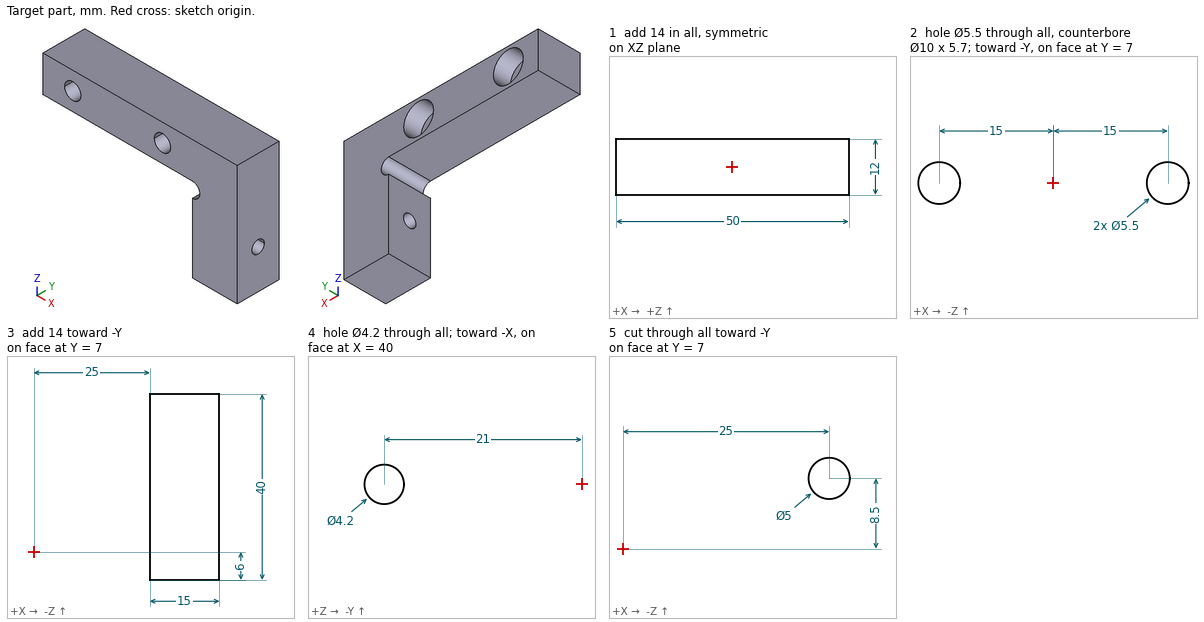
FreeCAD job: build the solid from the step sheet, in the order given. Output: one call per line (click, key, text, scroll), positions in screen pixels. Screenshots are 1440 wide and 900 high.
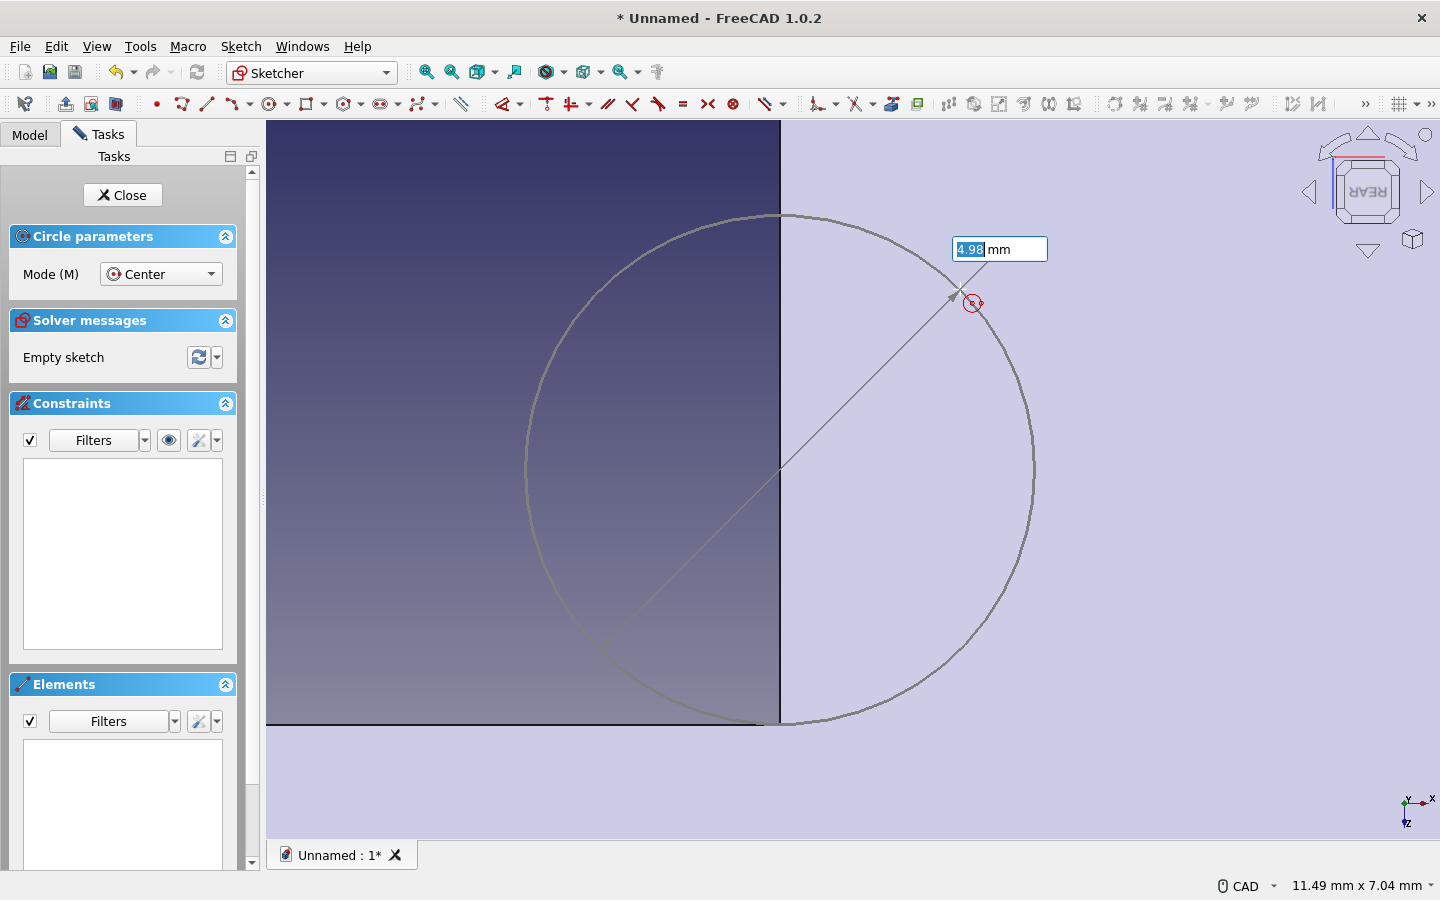
text(5)
key(Return)
key(Escape)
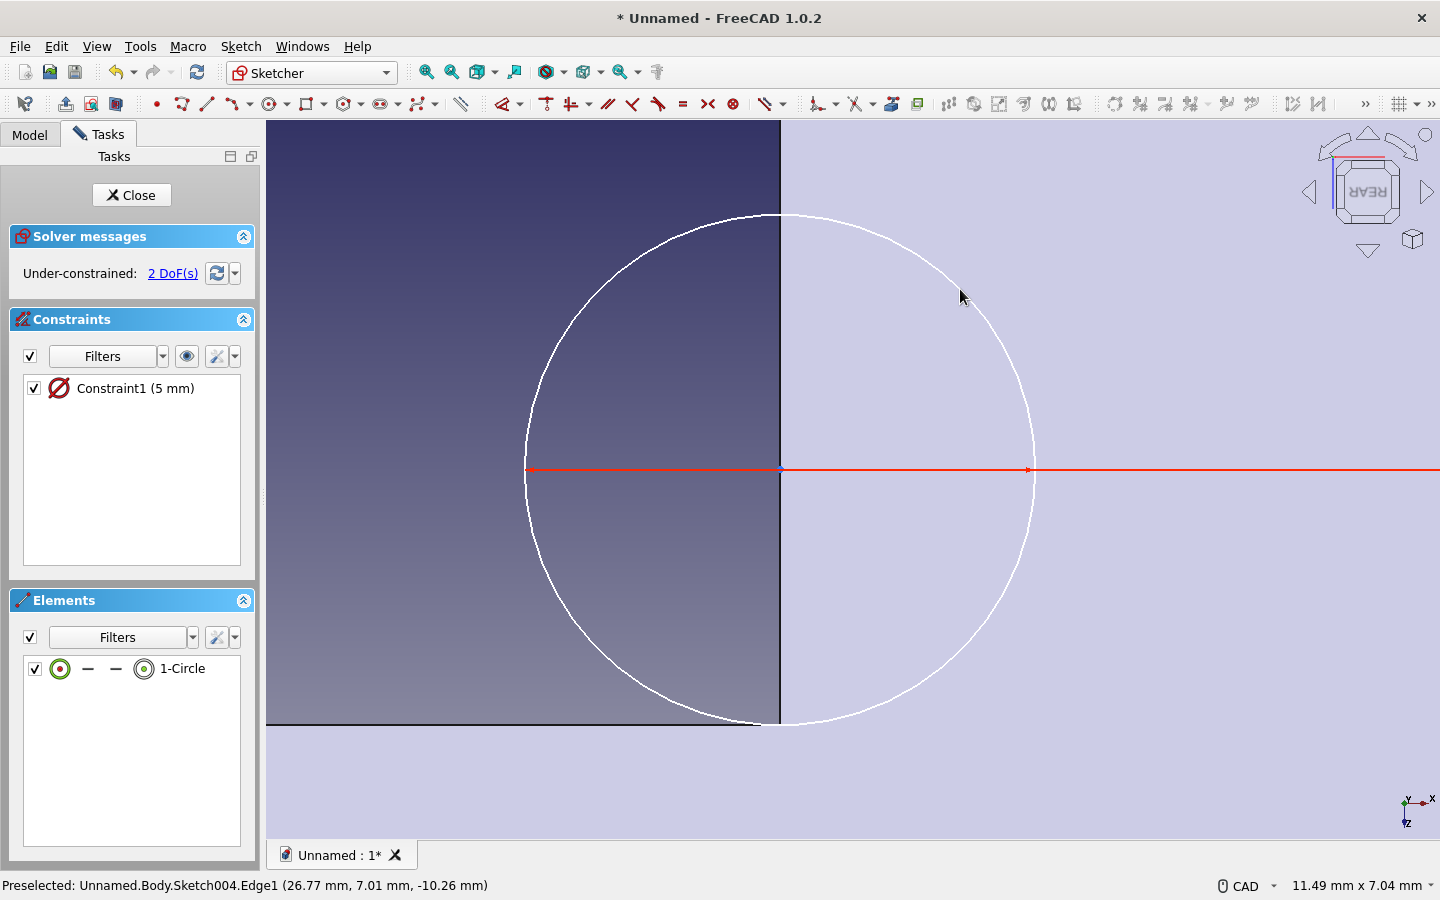
click(502, 104)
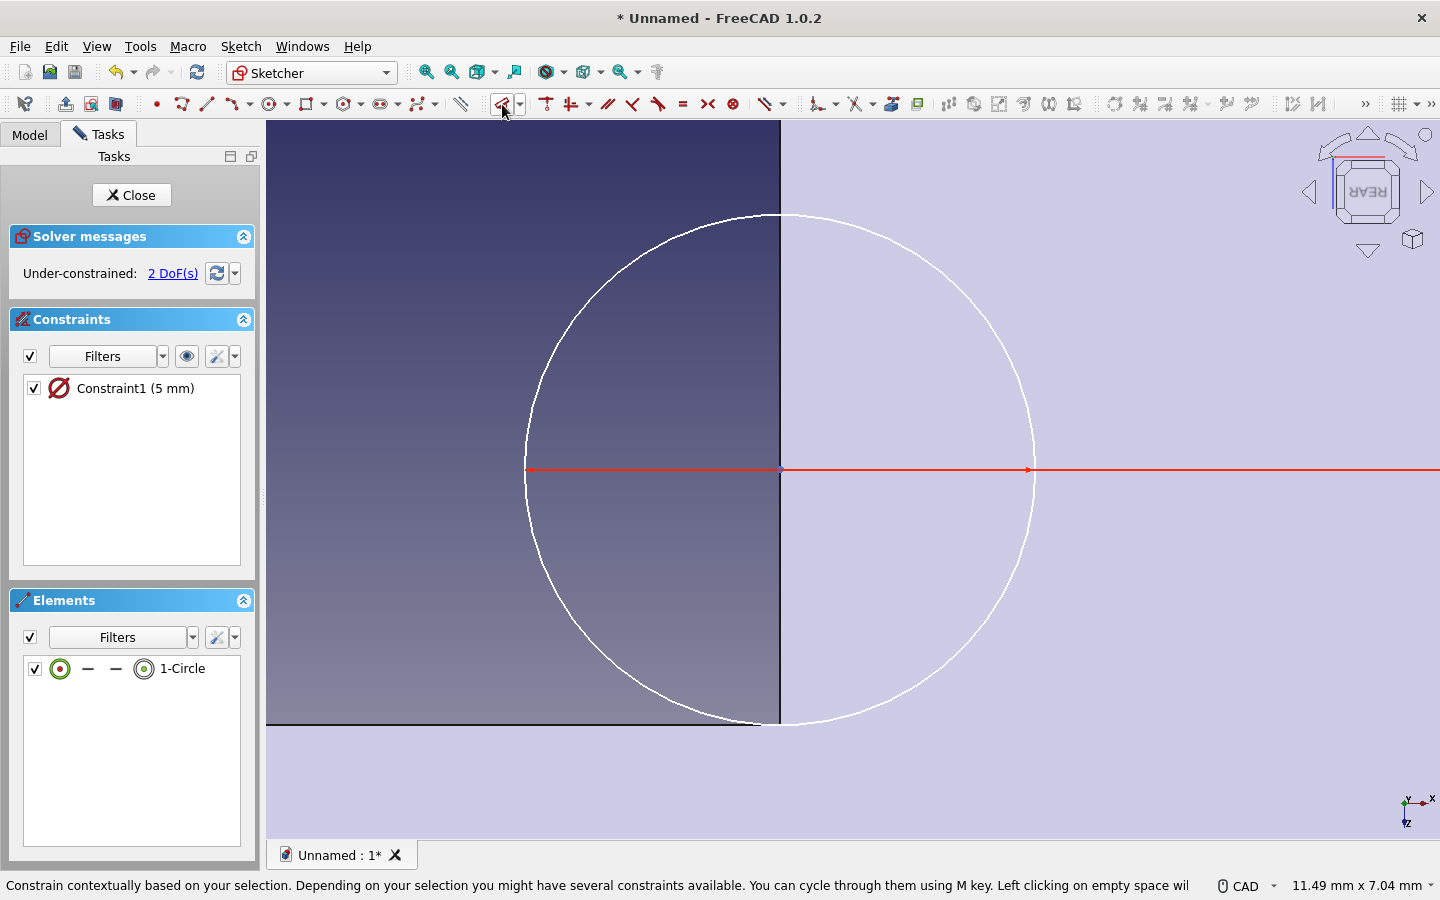
click(780, 470)
click(425, 436)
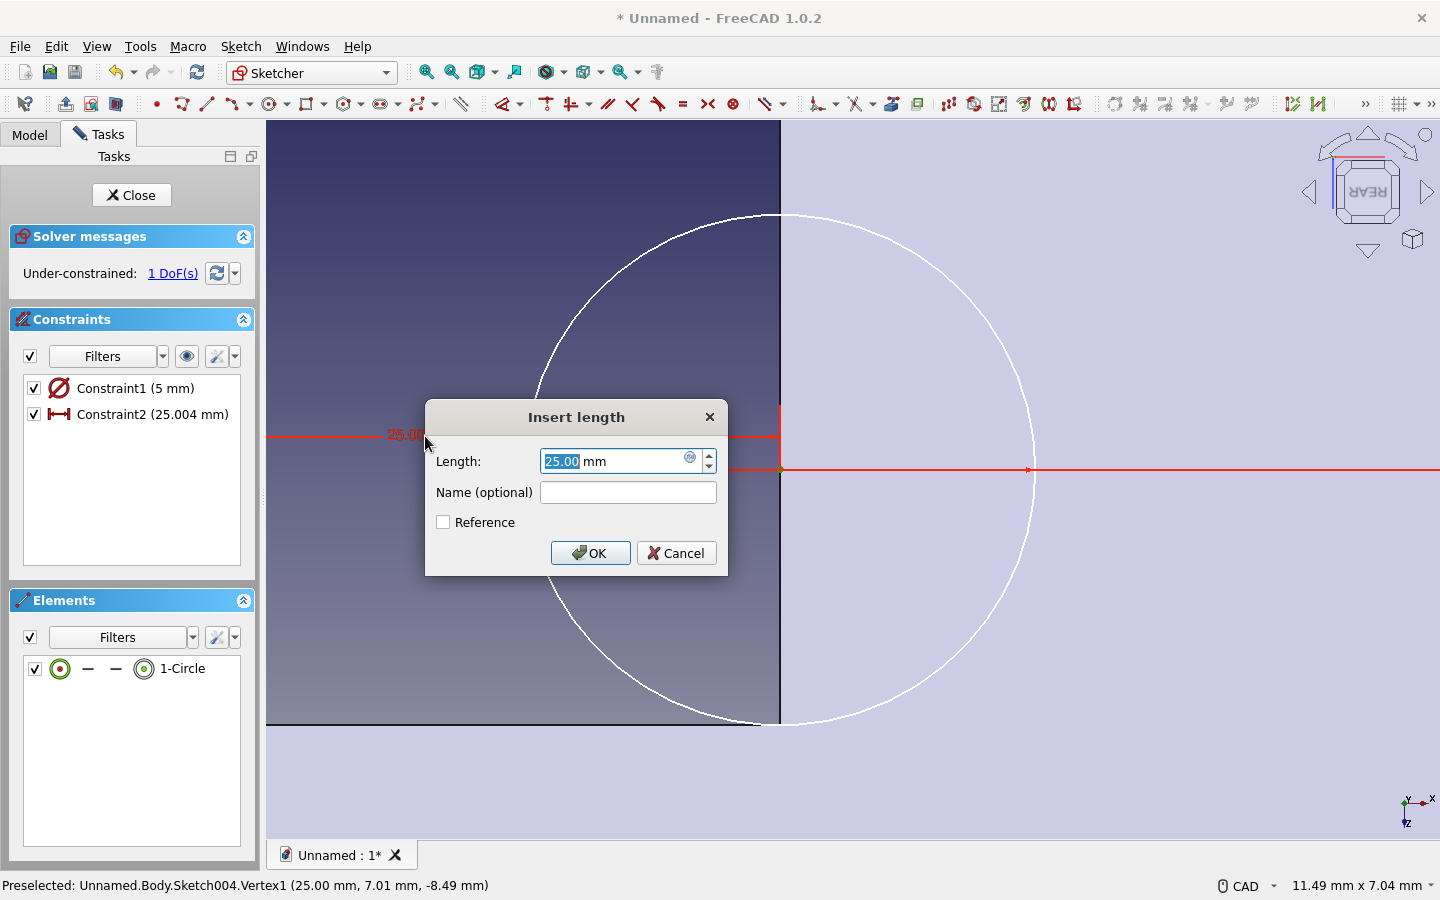
text(25)
key(Return)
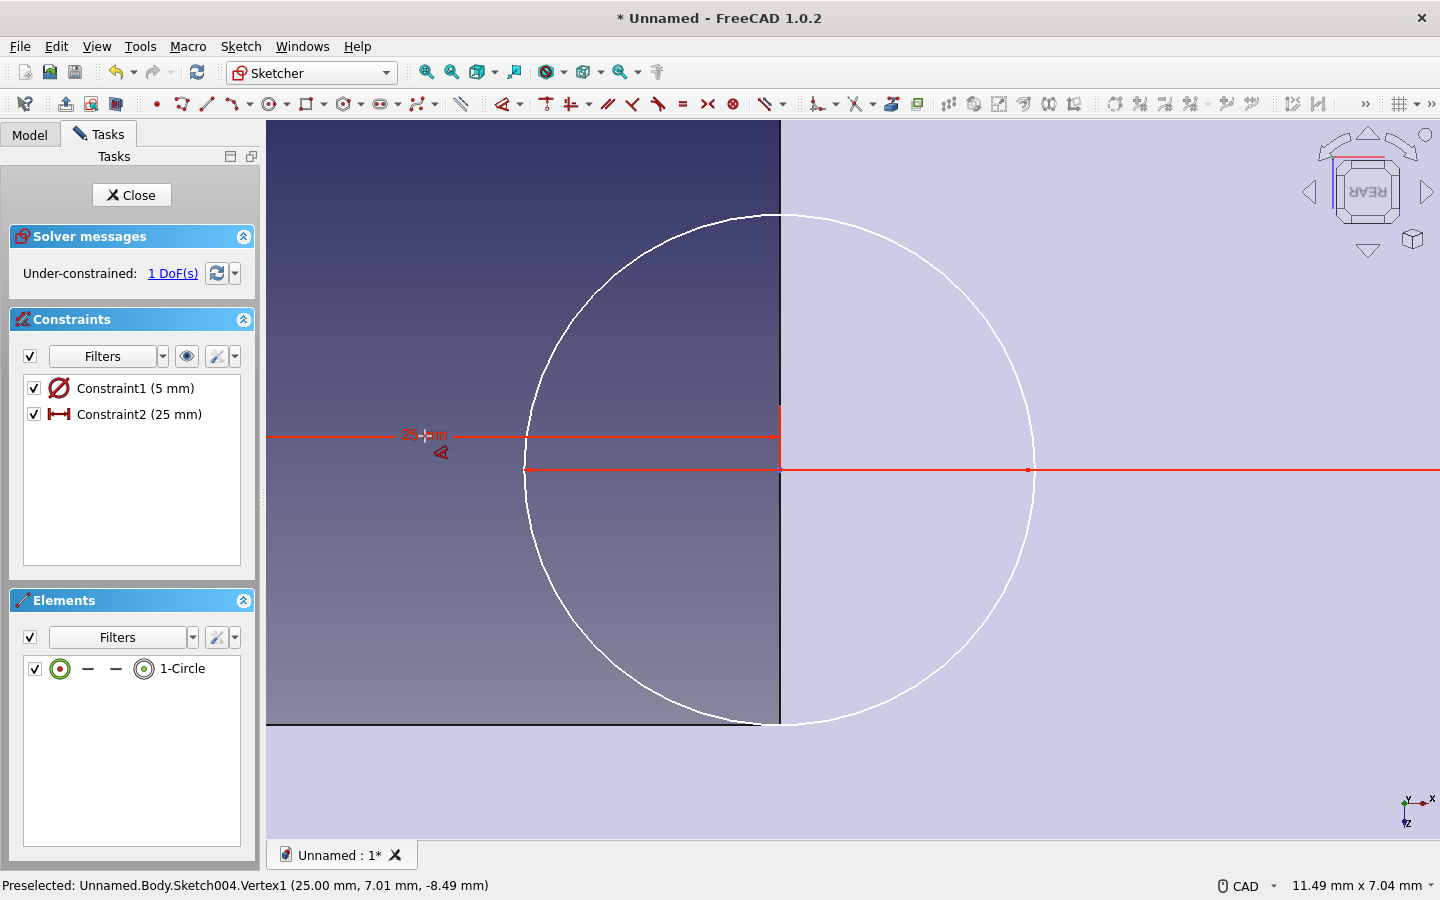
click(780, 470)
click(814, 641)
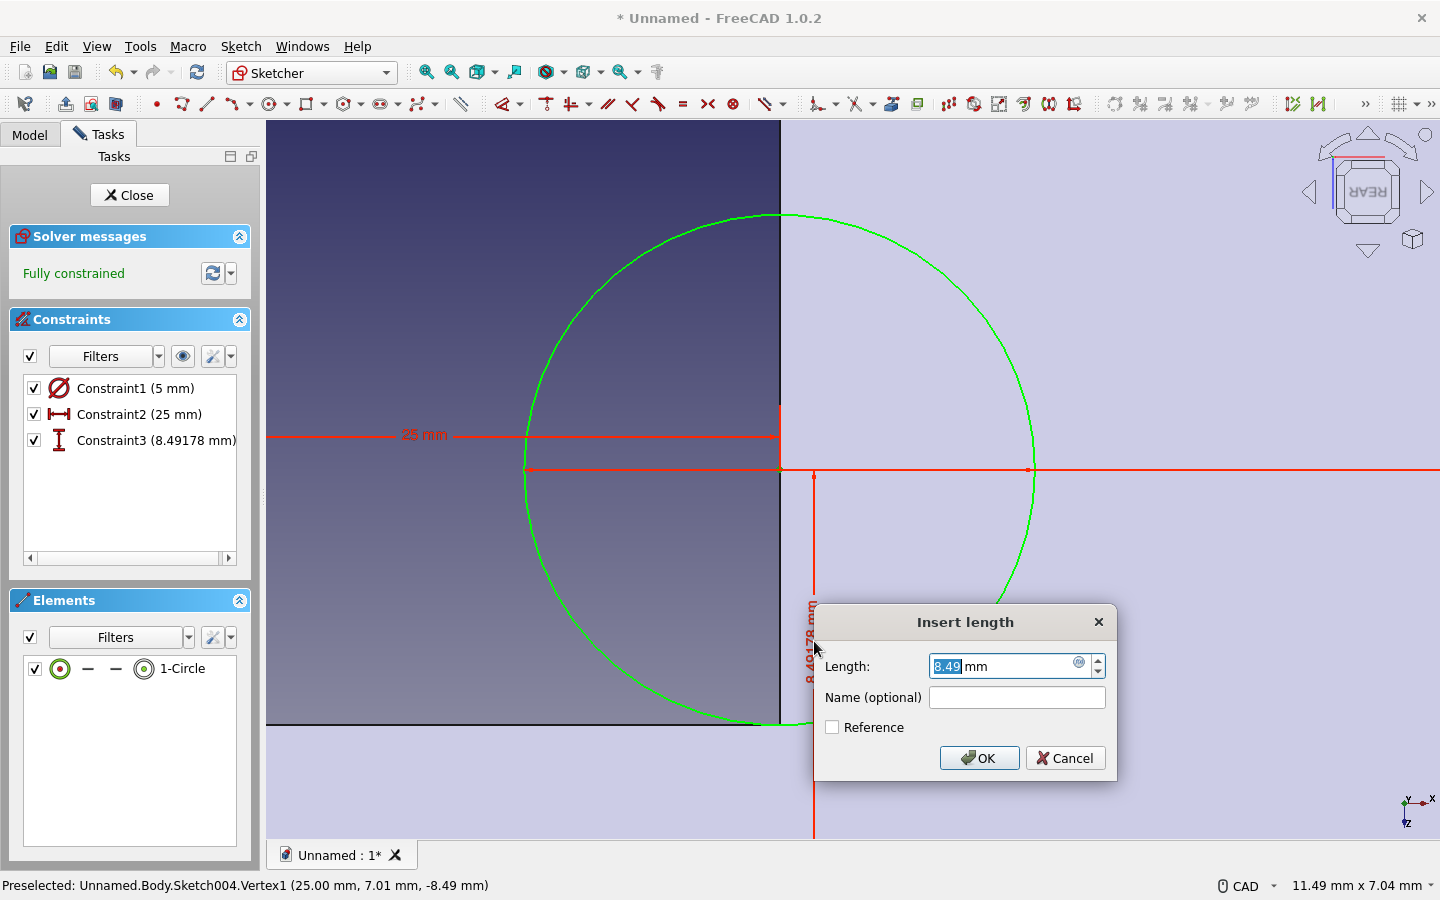
text(8.5)
key(Return)
key(Escape)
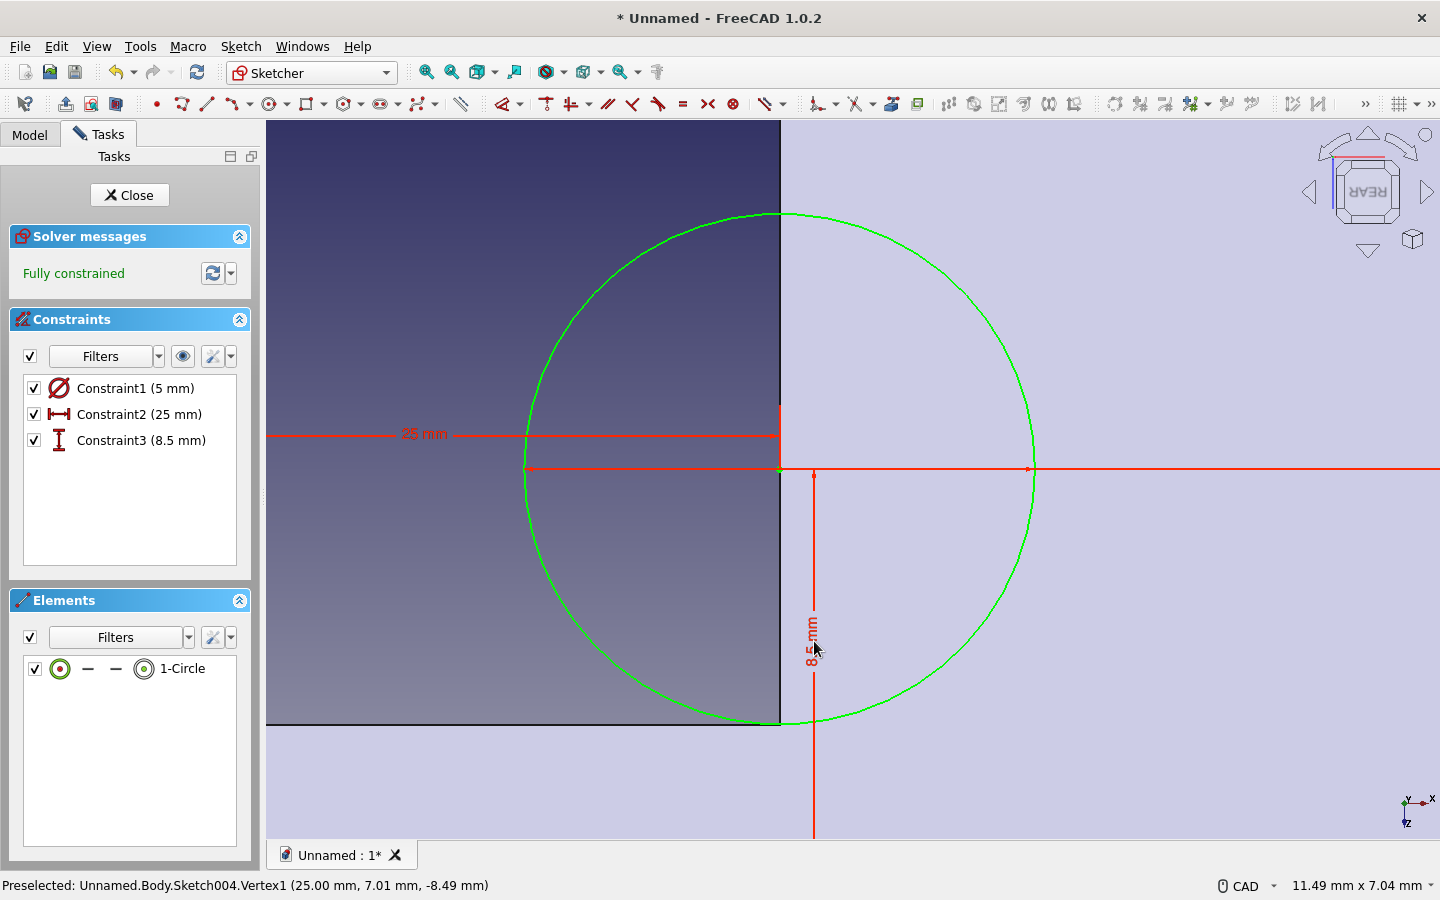
click(130, 195)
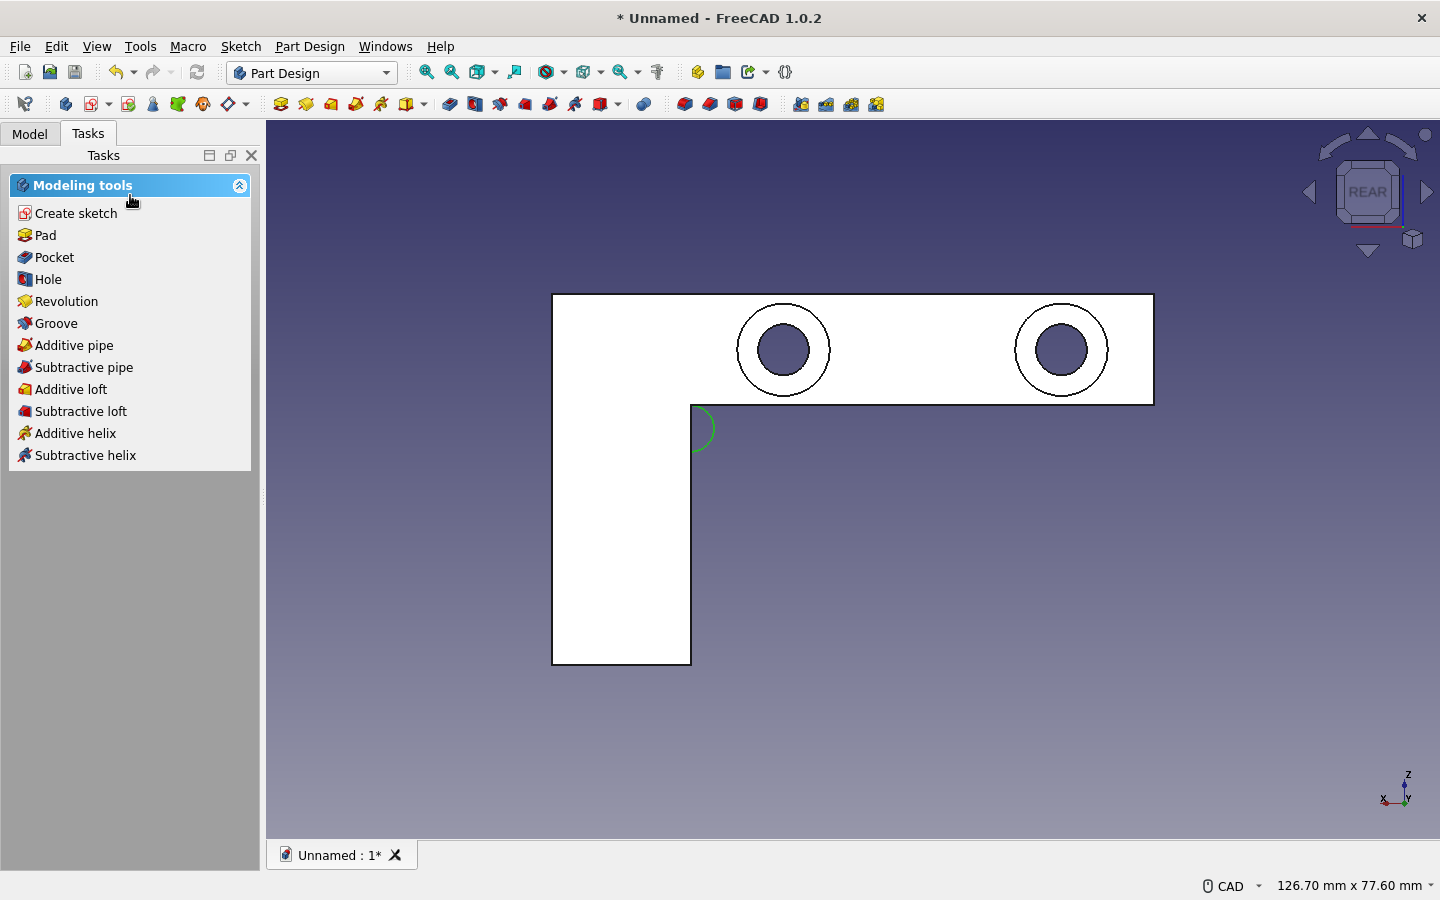
click(450, 104)